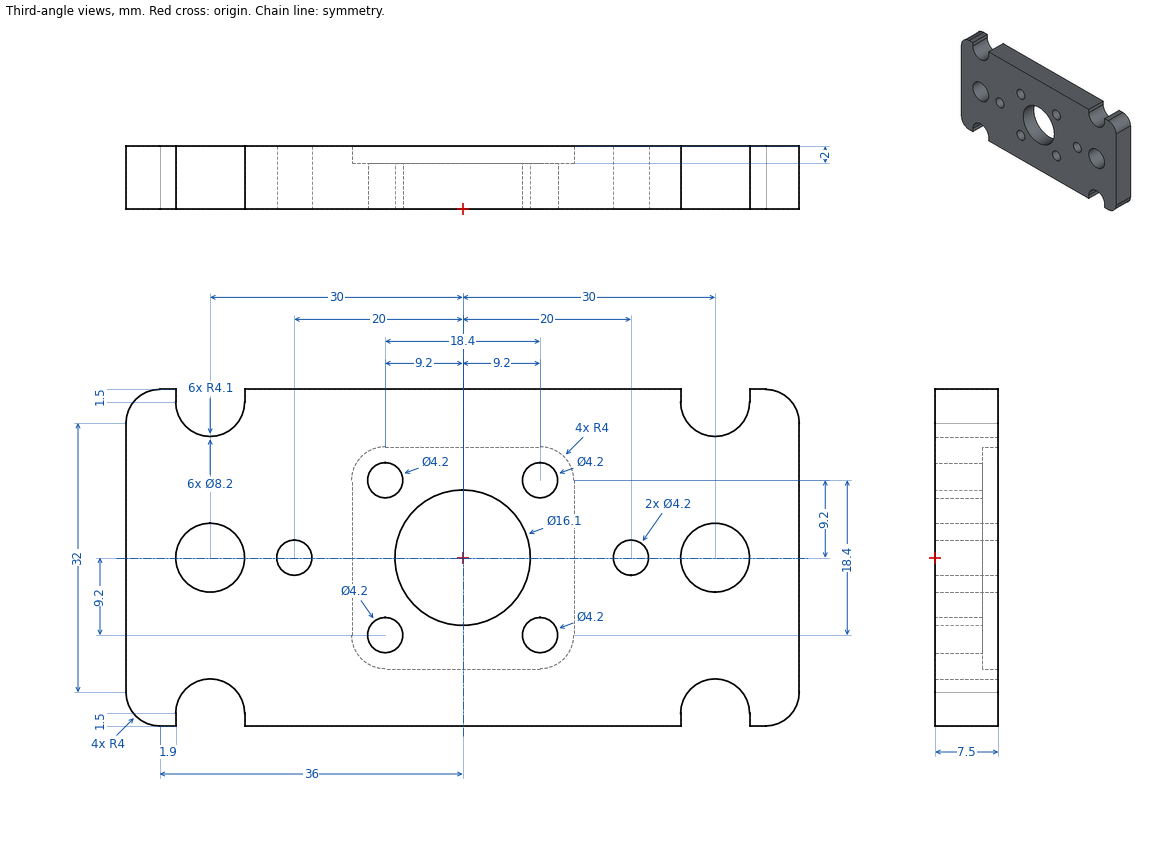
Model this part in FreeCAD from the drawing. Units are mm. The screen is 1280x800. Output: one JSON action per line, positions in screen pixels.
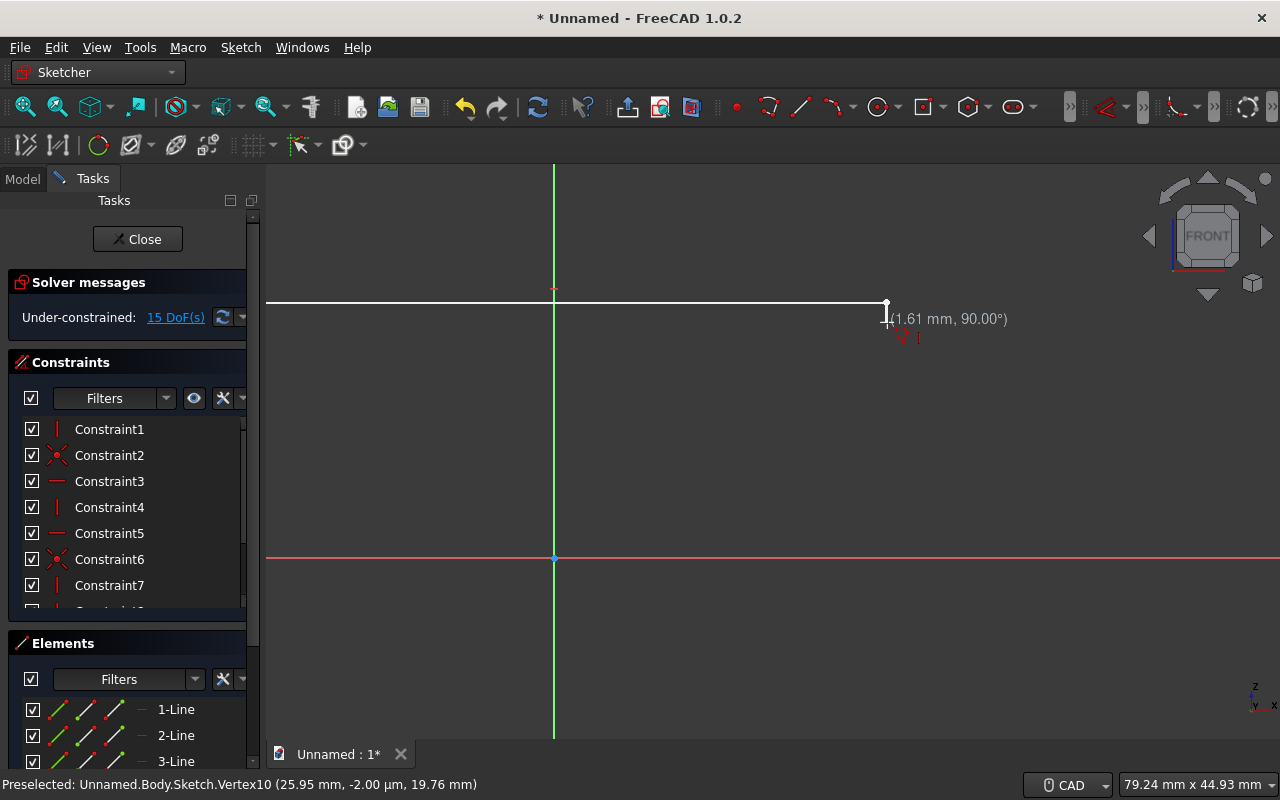
{"action": "left_click", "coordinate": [886, 321]}
{"action": "right_click", "coordinate": [886, 321]}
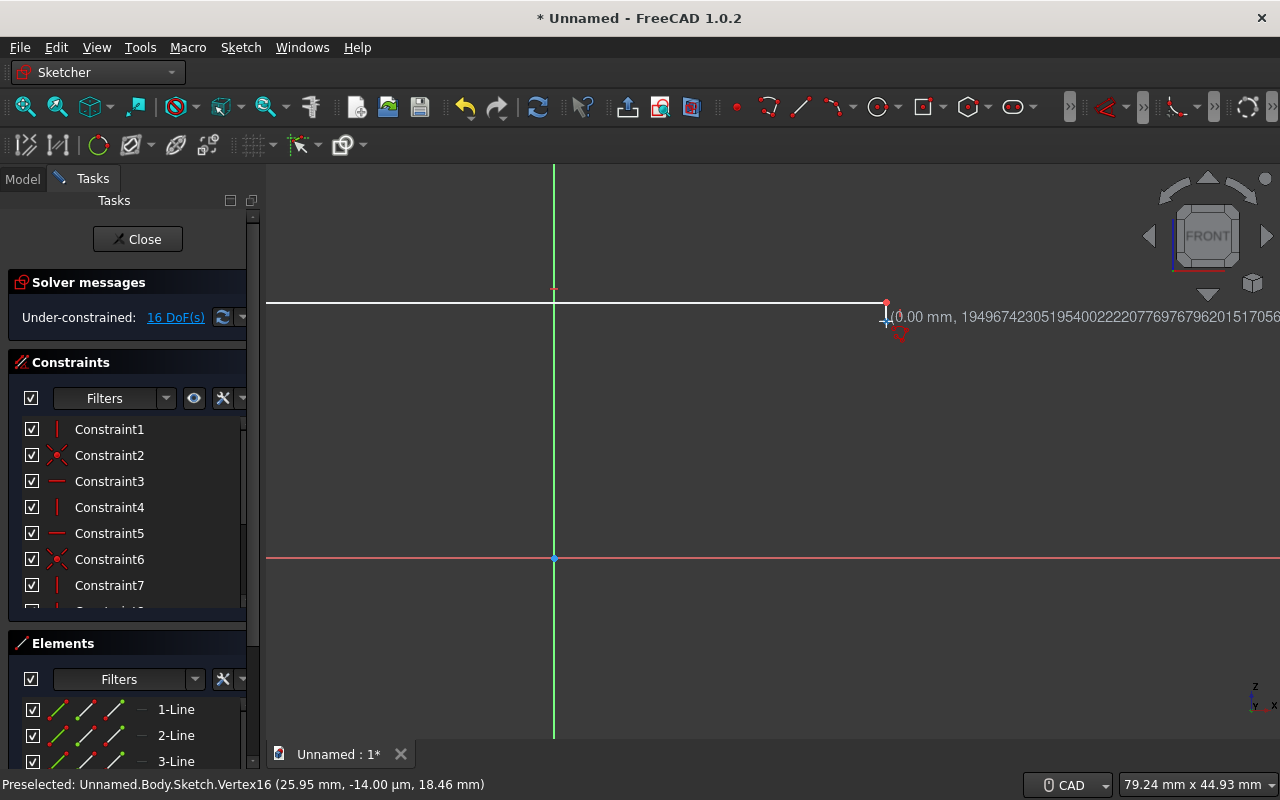
{"action": "left_click", "coordinate": [991, 321]}
{"action": "left_click", "coordinate": [991, 302]}
{"action": "left_click", "coordinate": [1015, 302]}
{"action": "right_click", "coordinate": [1015, 302]}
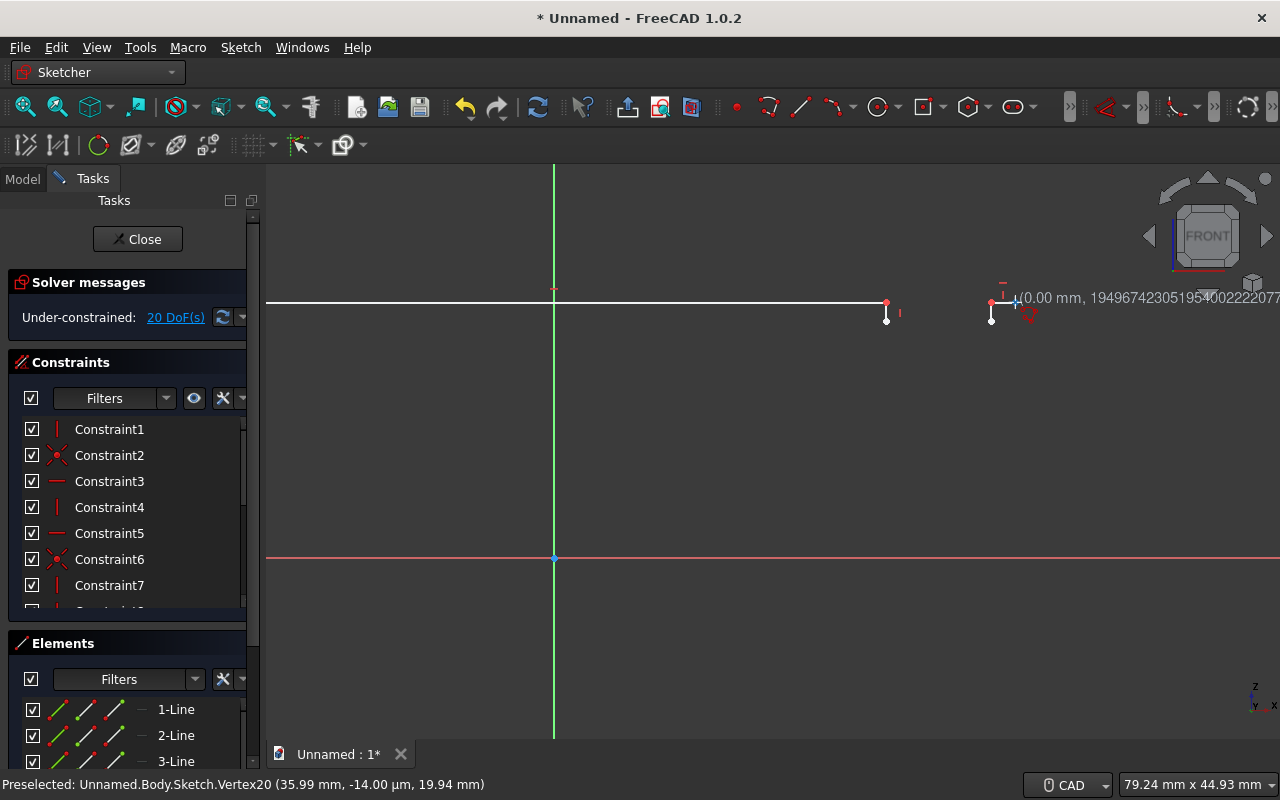
{"action": "left_click", "coordinate": [802, 108]}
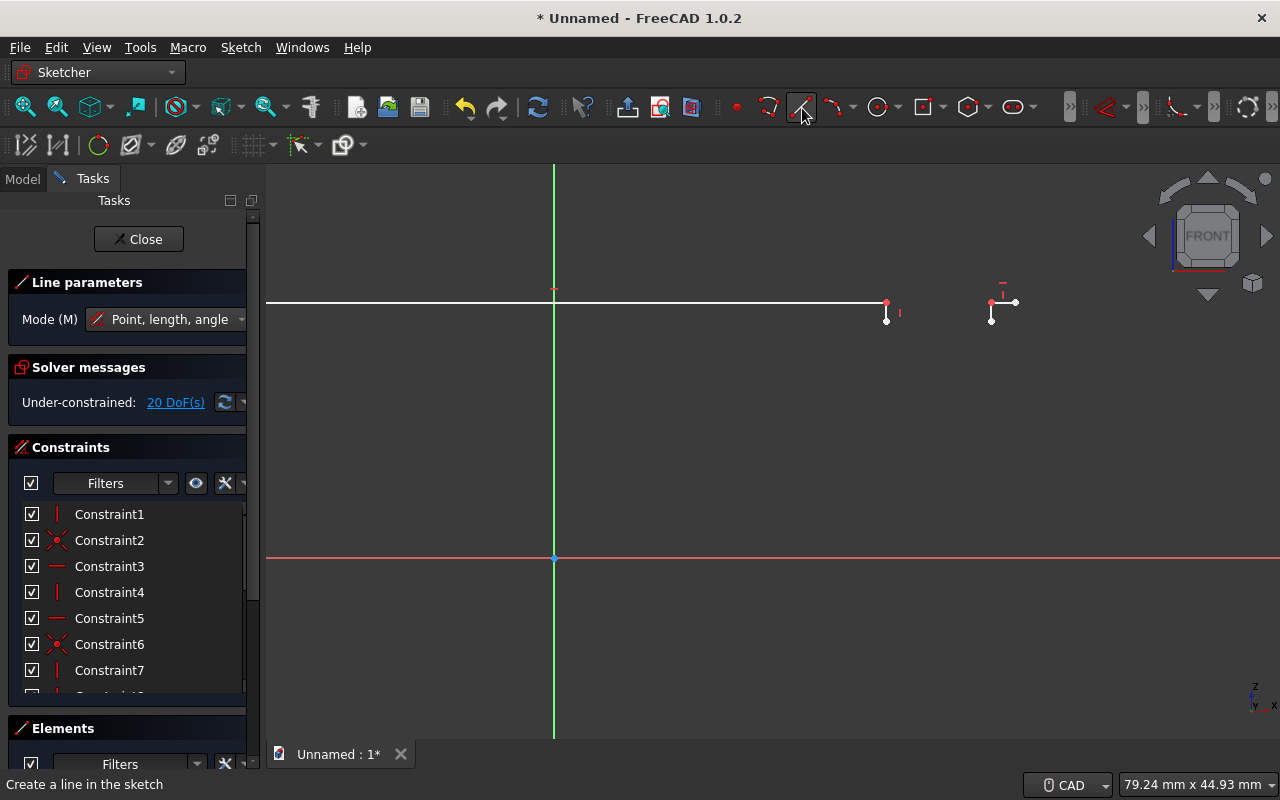
{"action": "left_click", "coordinate": [1066, 353]}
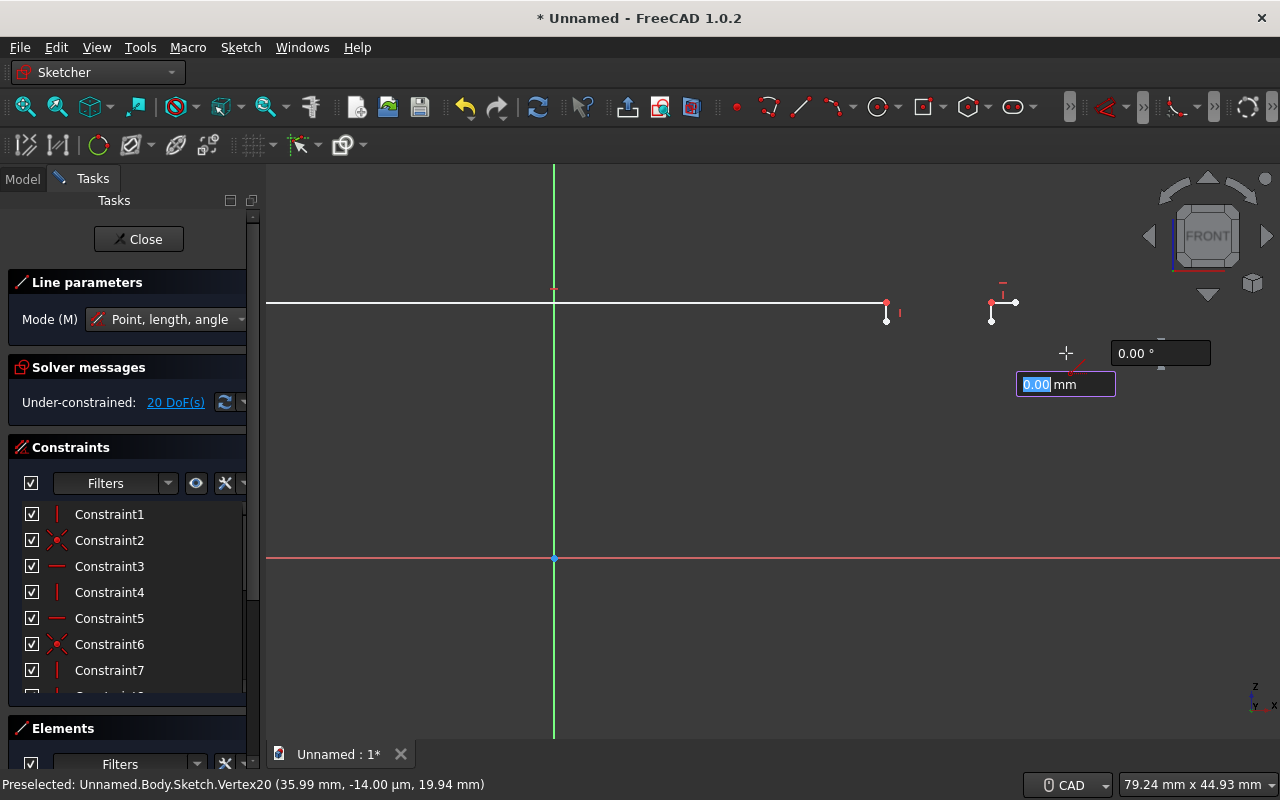
{"action": "scroll", "coordinate": [887, 322], "scroll_direction": "down", "scroll_amount": 3}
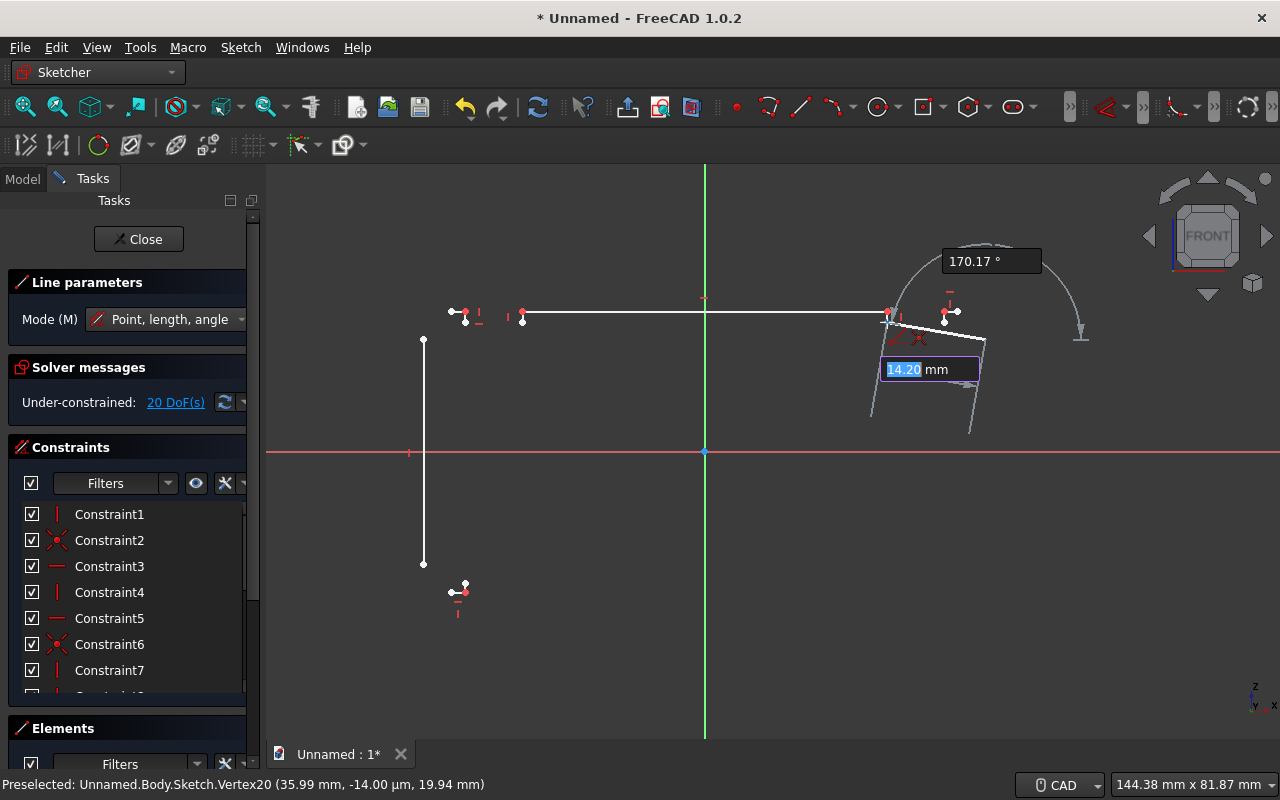
{"action": "left_click", "coordinate": [986, 564]}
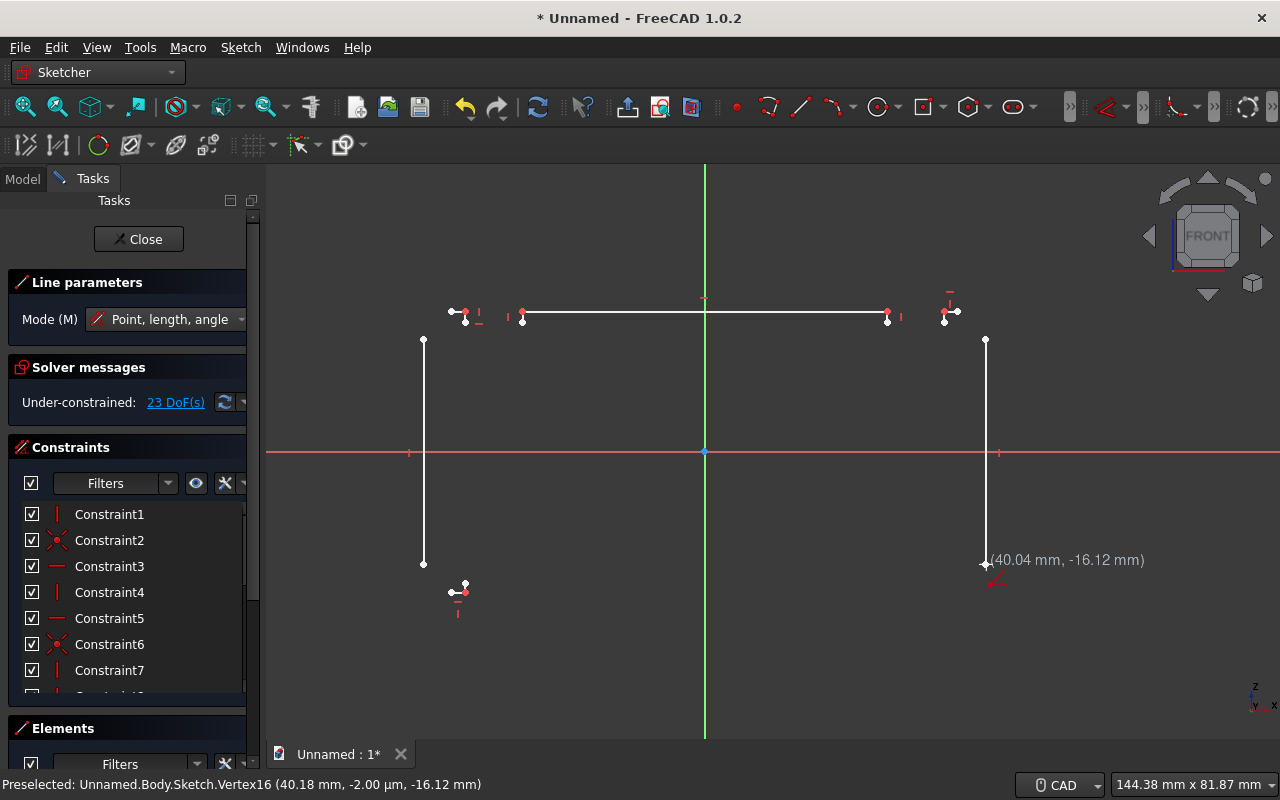
{"action": "left_click", "coordinate": [770, 108]}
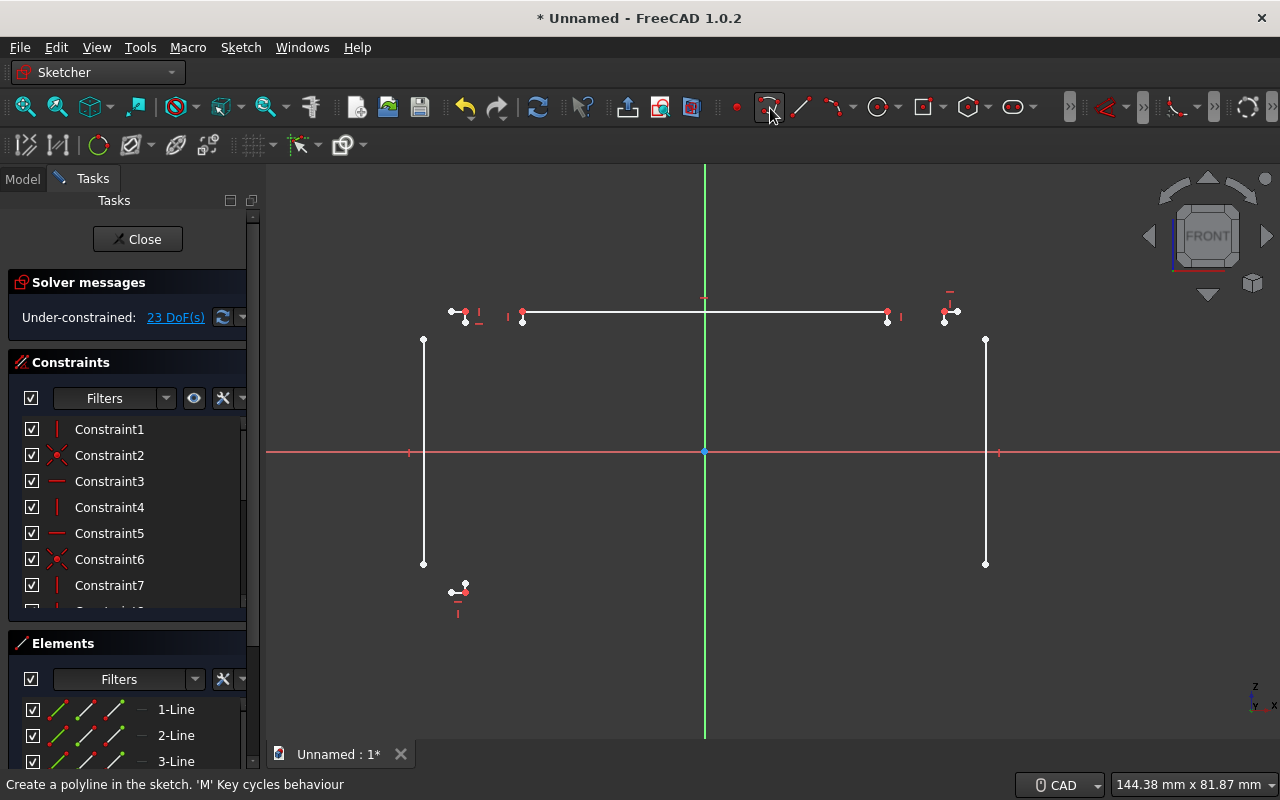
{"action": "left_click", "coordinate": [958, 592]}
{"action": "left_click", "coordinate": [944, 592]}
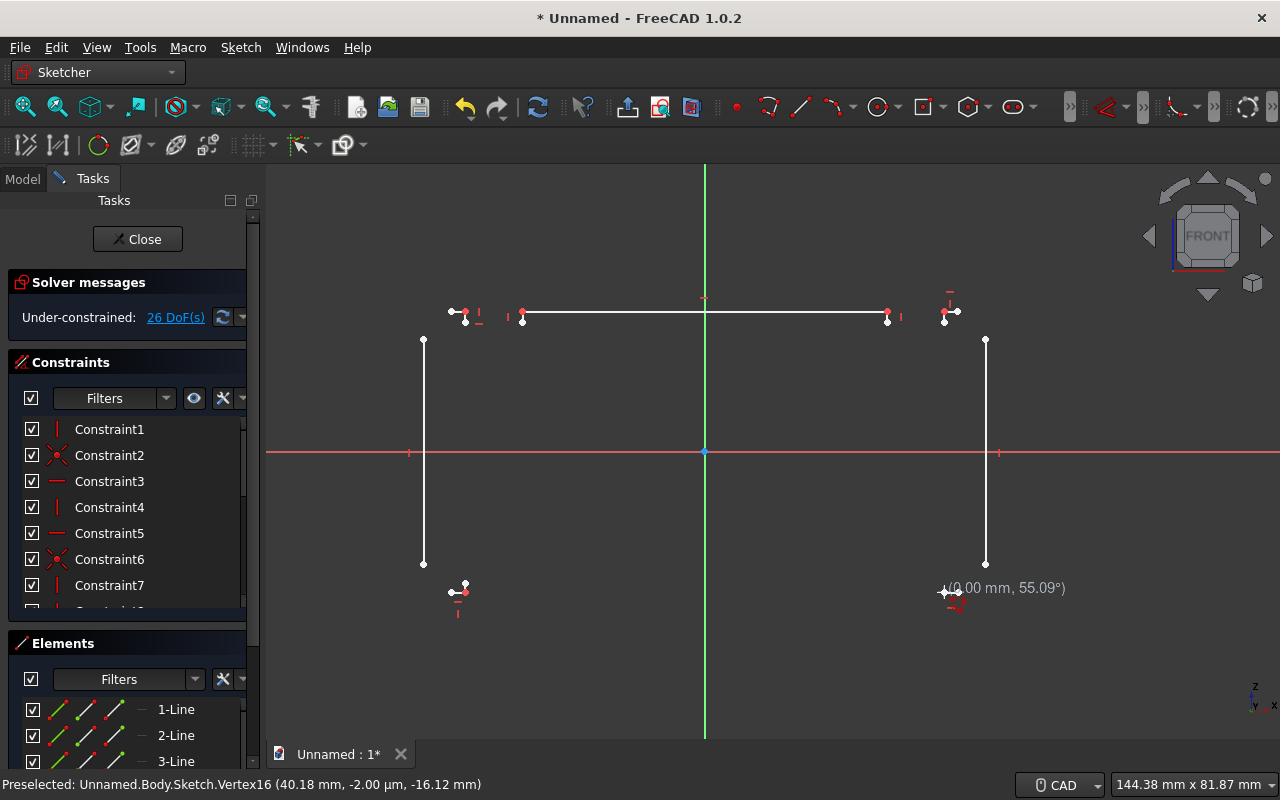
{"action": "scroll", "coordinate": [944, 582], "scroll_direction": "up", "scroll_amount": 3}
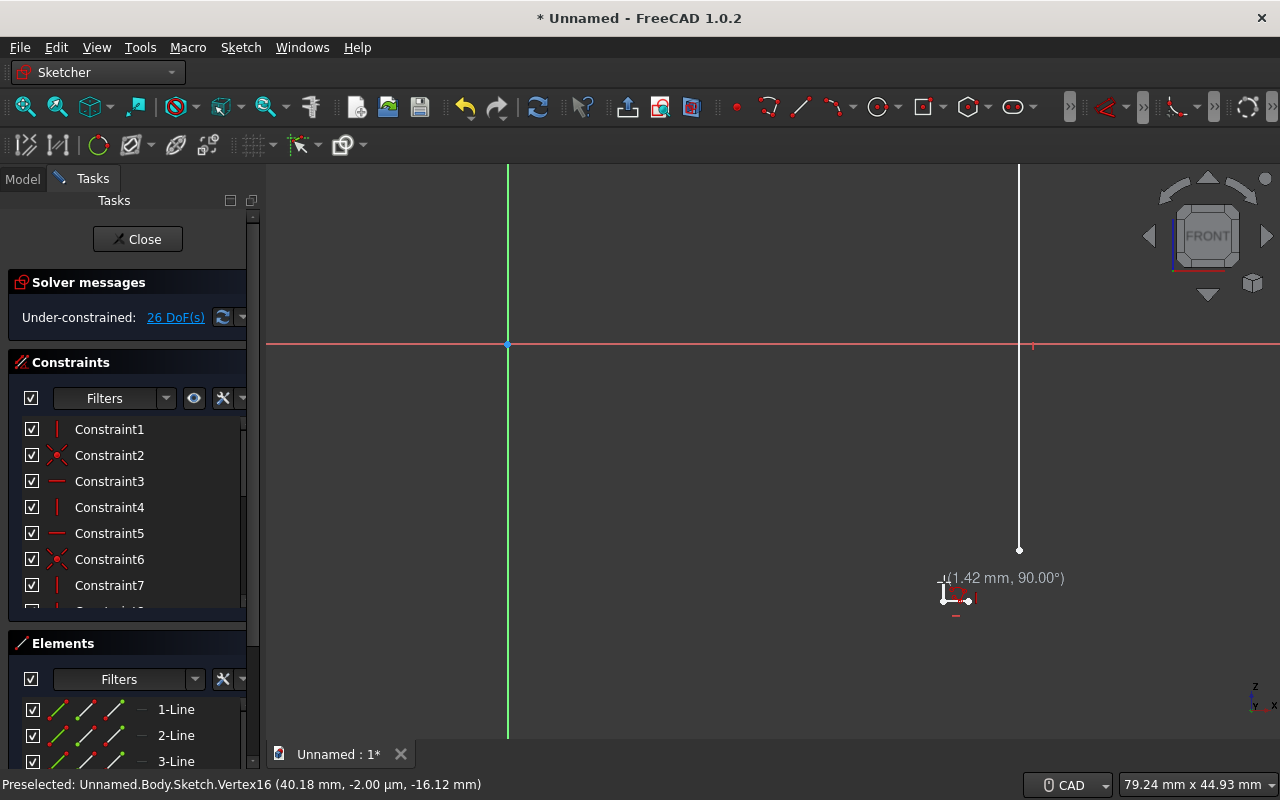
{"action": "left_click", "coordinate": [943, 581]}
{"action": "right_click", "coordinate": [943, 581]}